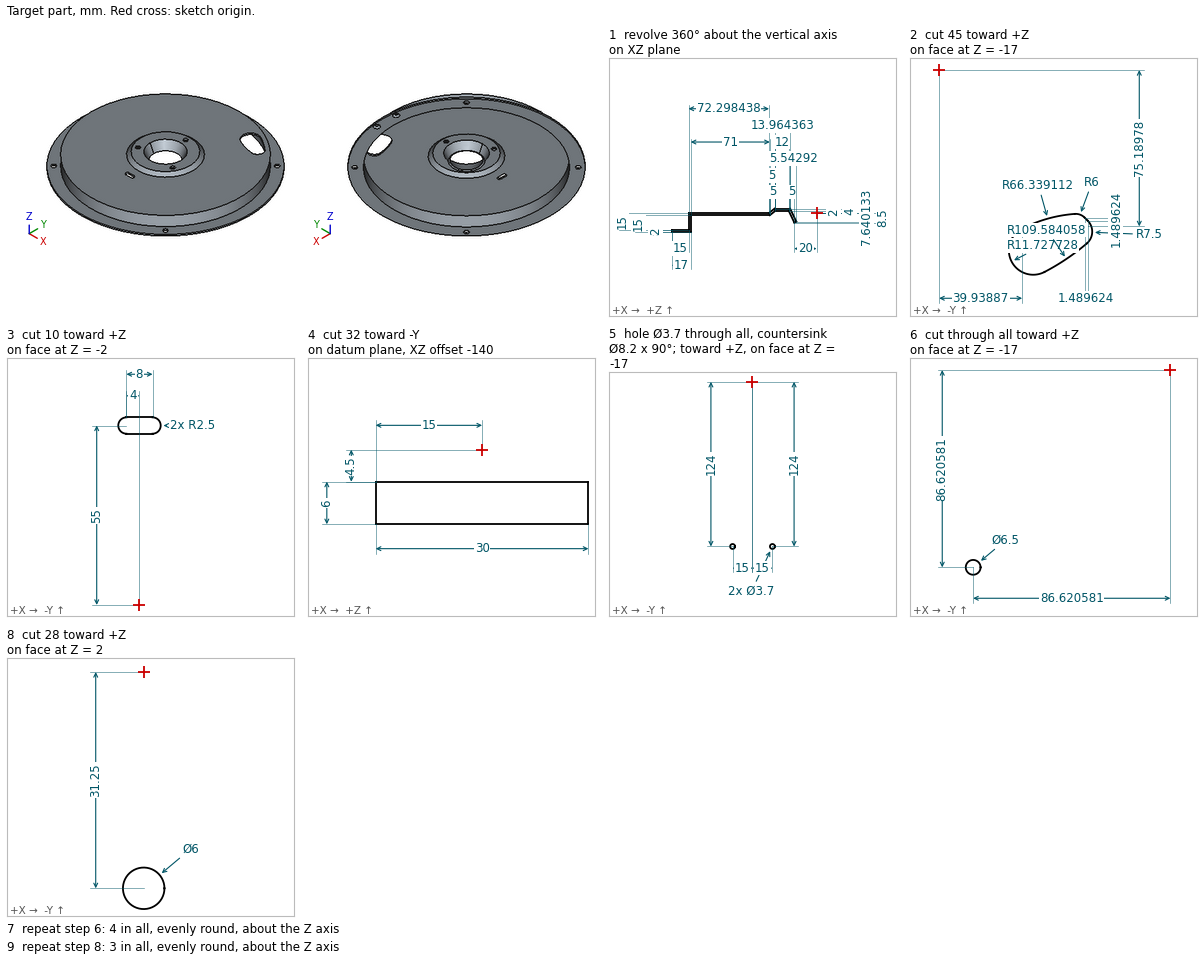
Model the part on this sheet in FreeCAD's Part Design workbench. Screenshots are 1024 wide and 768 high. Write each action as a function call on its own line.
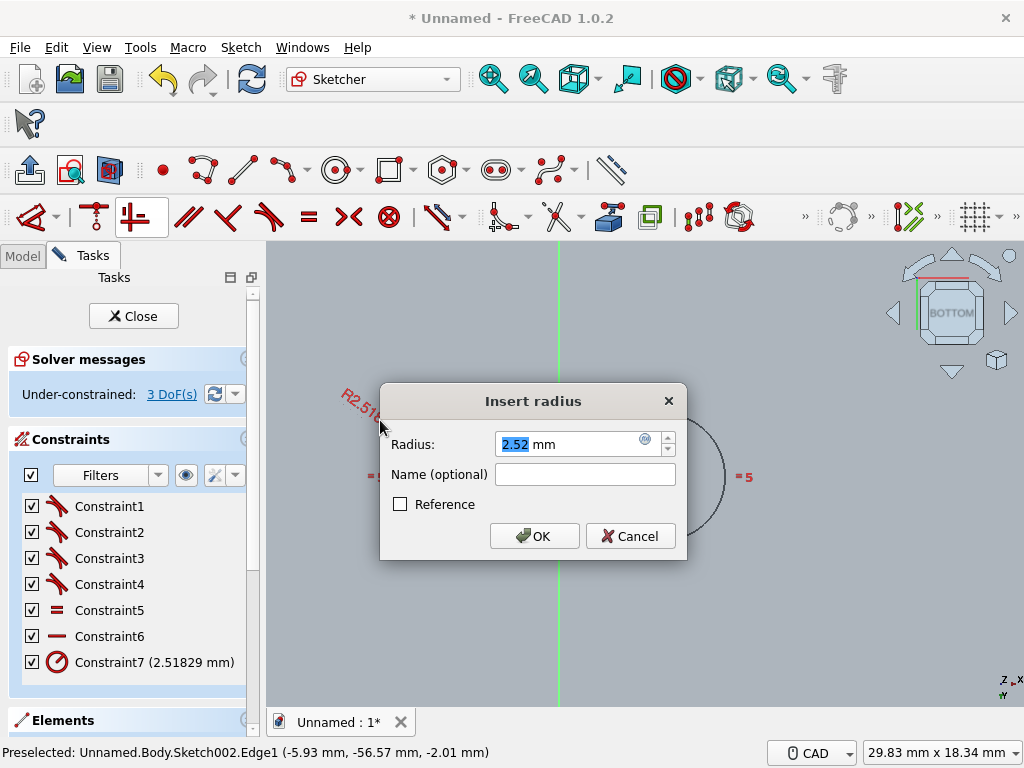
text(2.5)
key(Return)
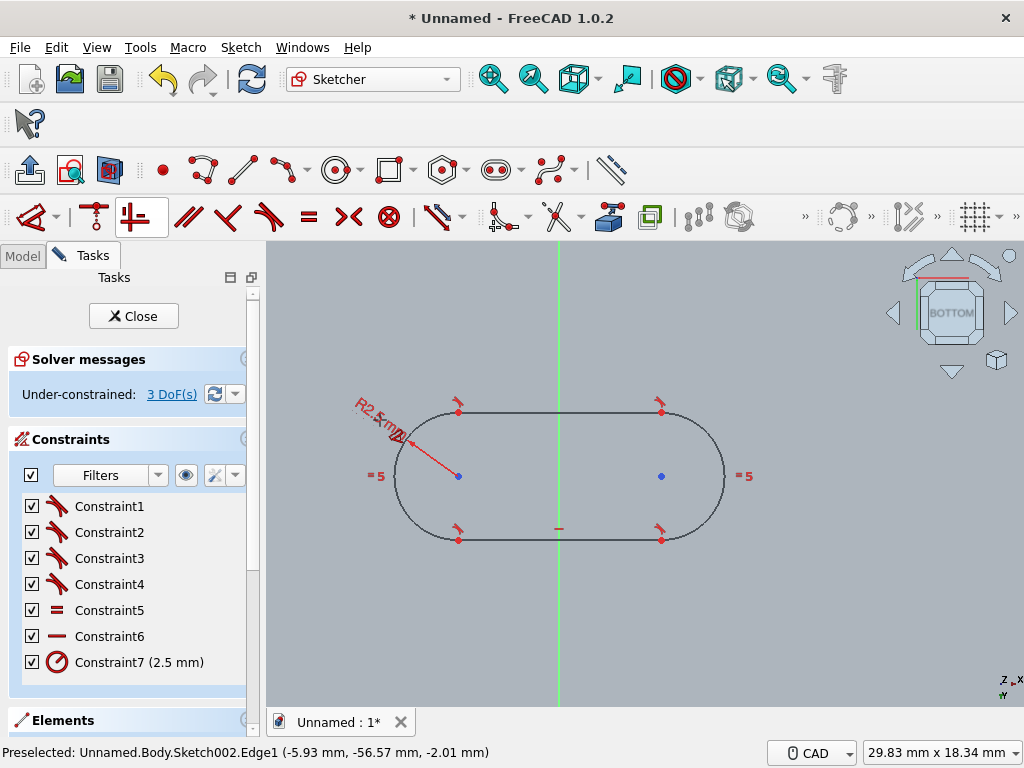
click(519, 413)
click(513, 379)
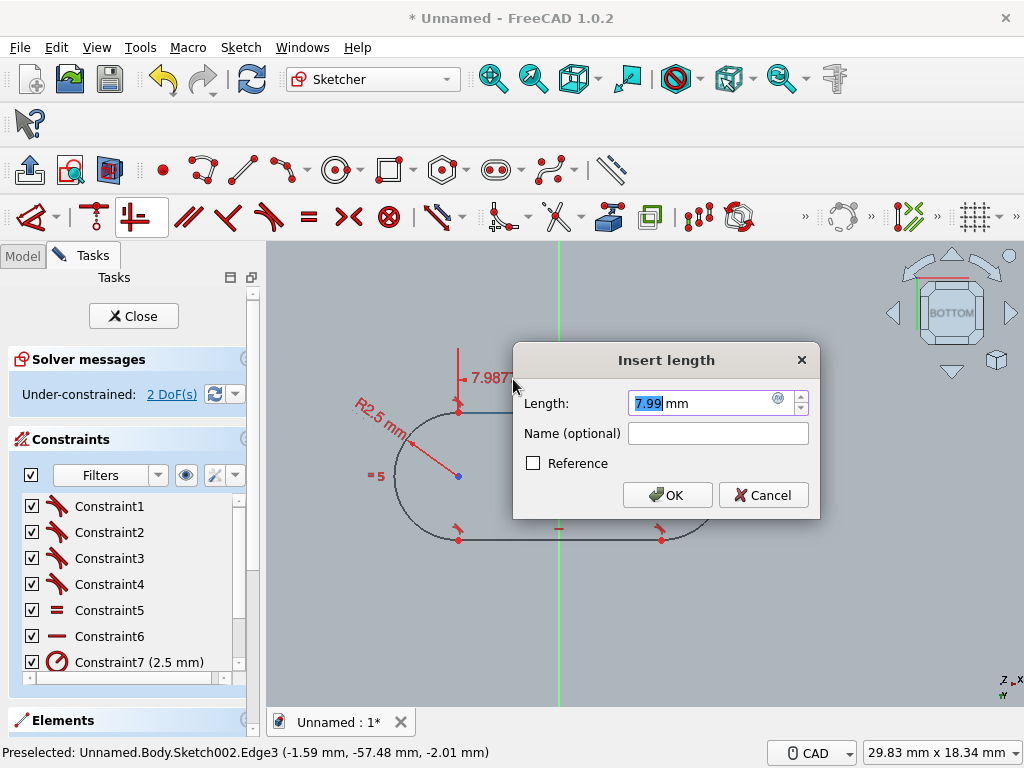
text(8)
key(Return)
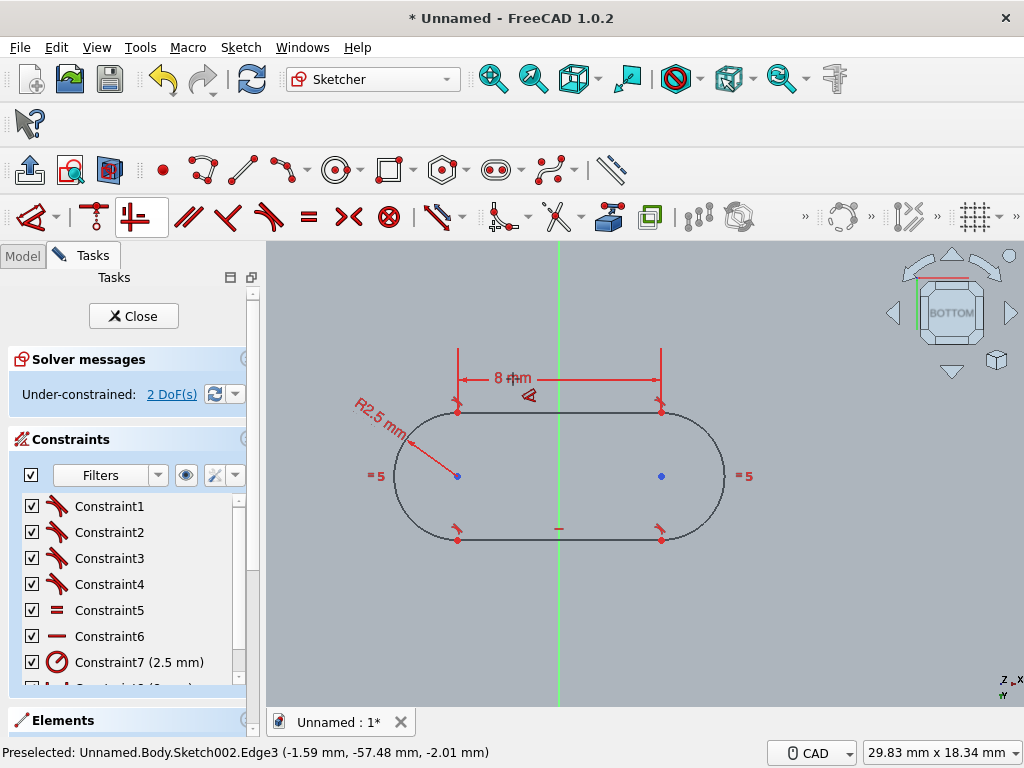
click(458, 413)
click(509, 355)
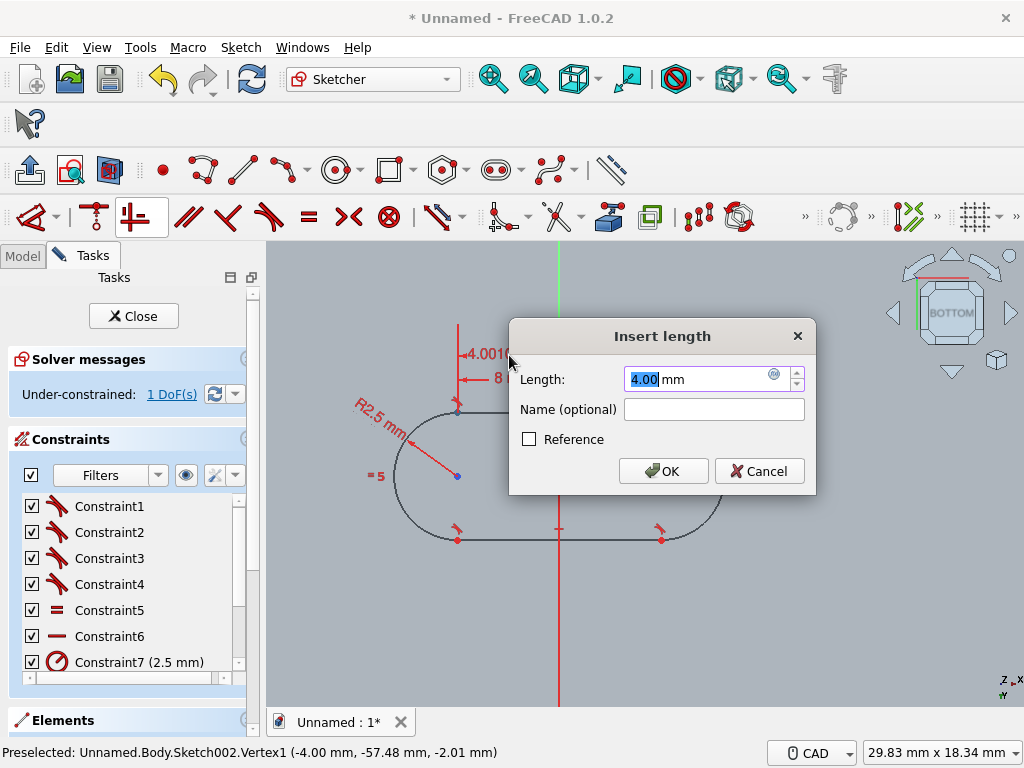
text(4)
key(Return)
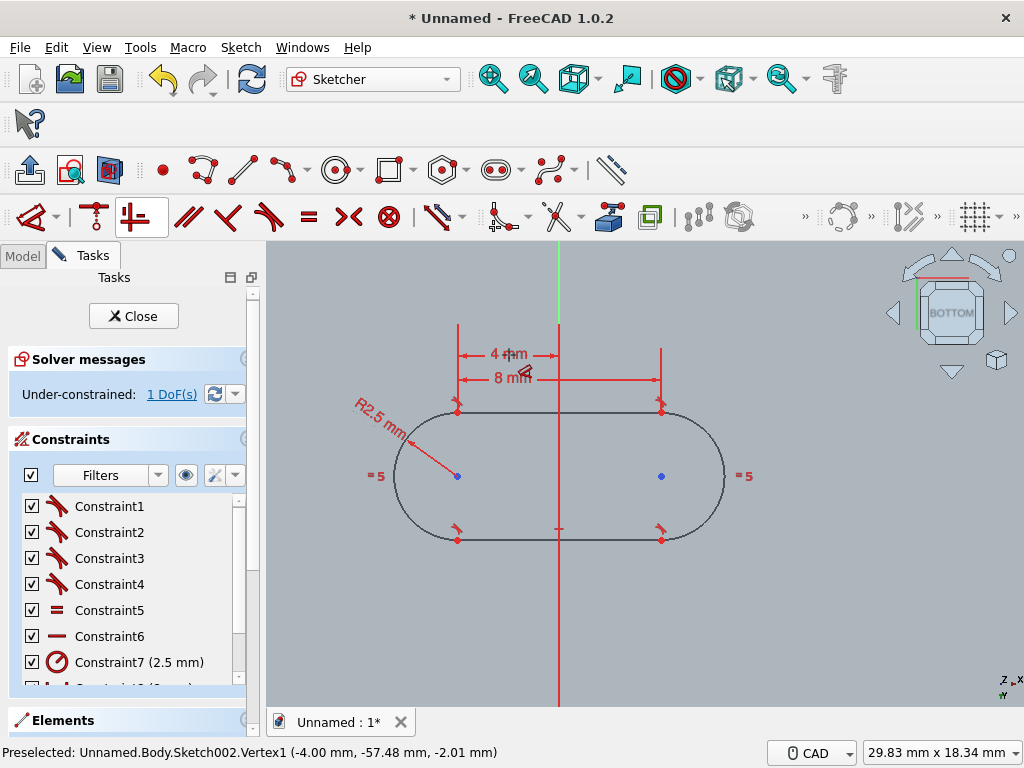
click(458, 477)
click(424, 578)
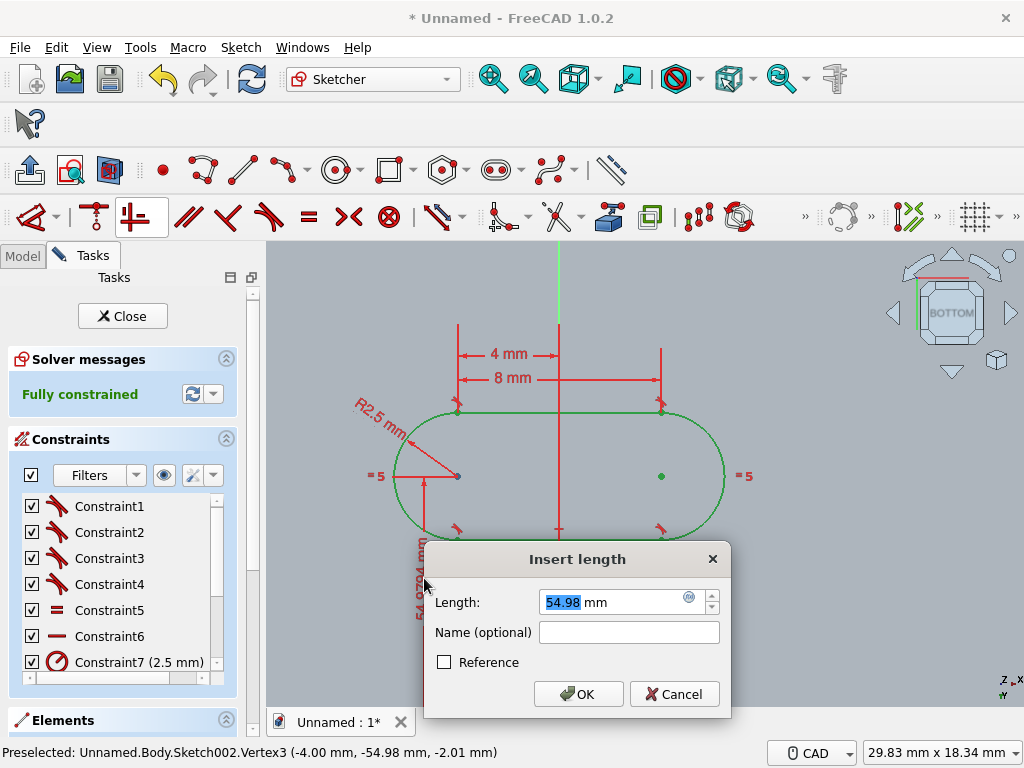
text(55)
key(Return)
key(Escape)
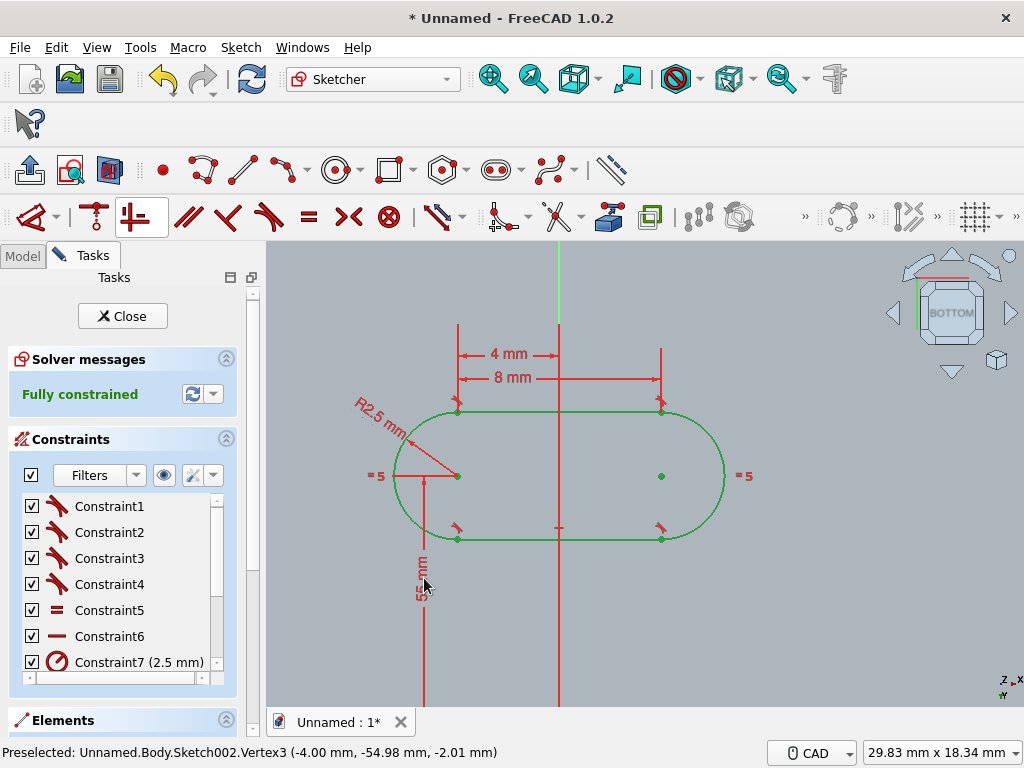
click(123, 316)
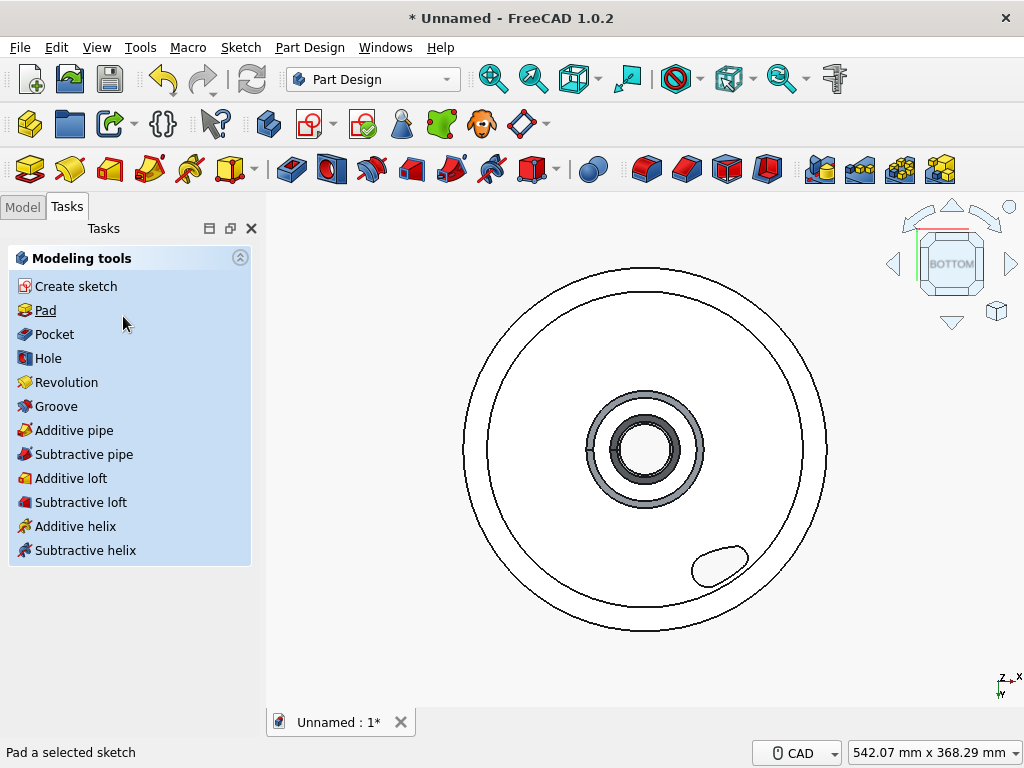
click(292, 170)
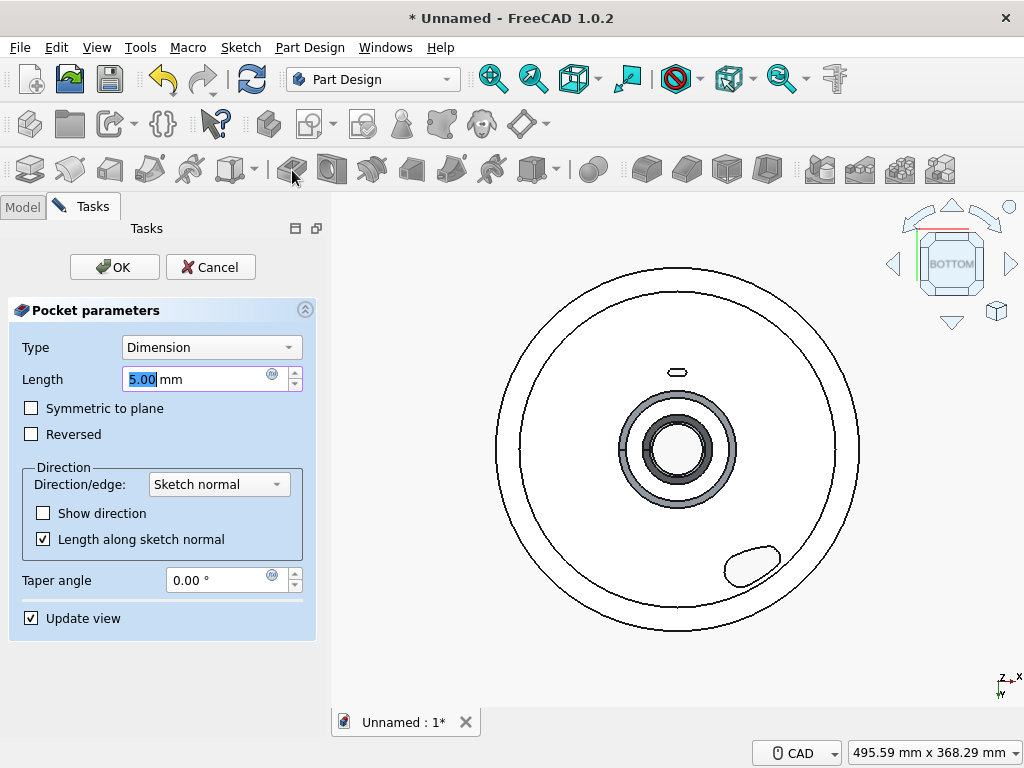
text(10)
key(Tab)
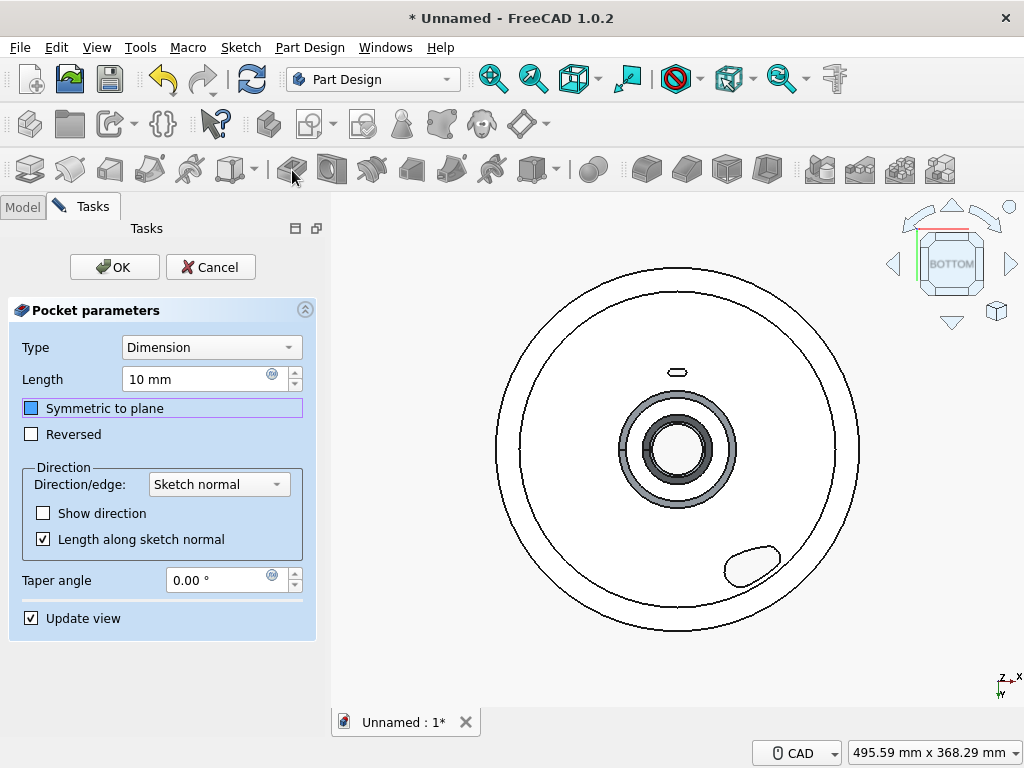
click(115, 267)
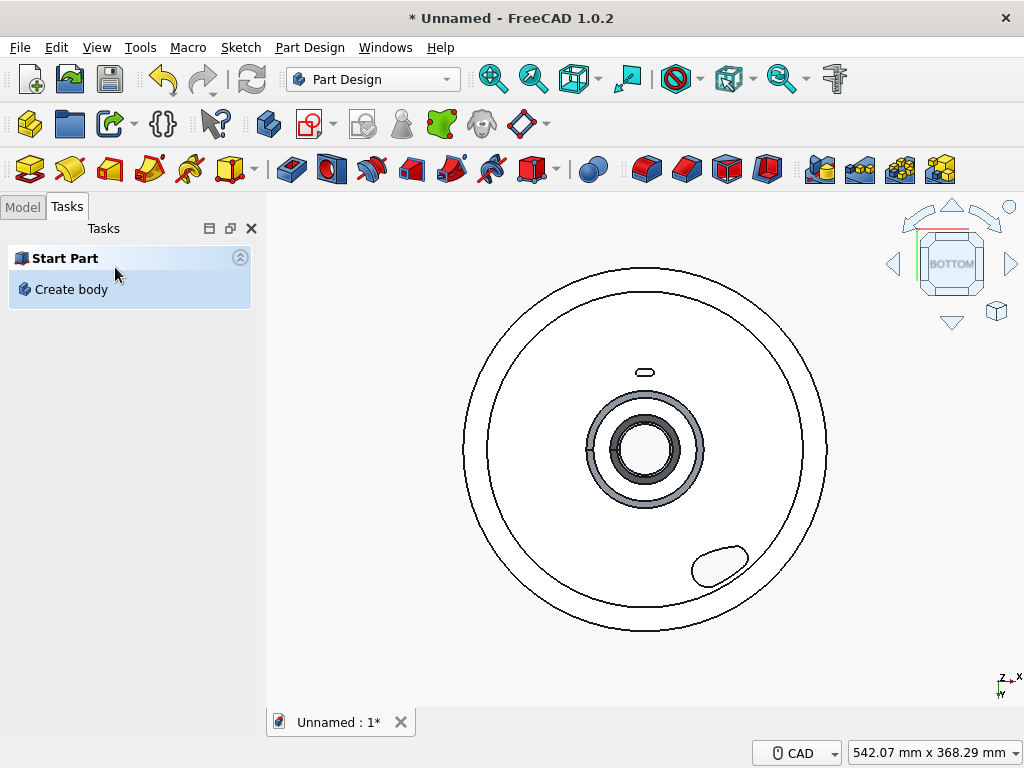
click(23, 206)